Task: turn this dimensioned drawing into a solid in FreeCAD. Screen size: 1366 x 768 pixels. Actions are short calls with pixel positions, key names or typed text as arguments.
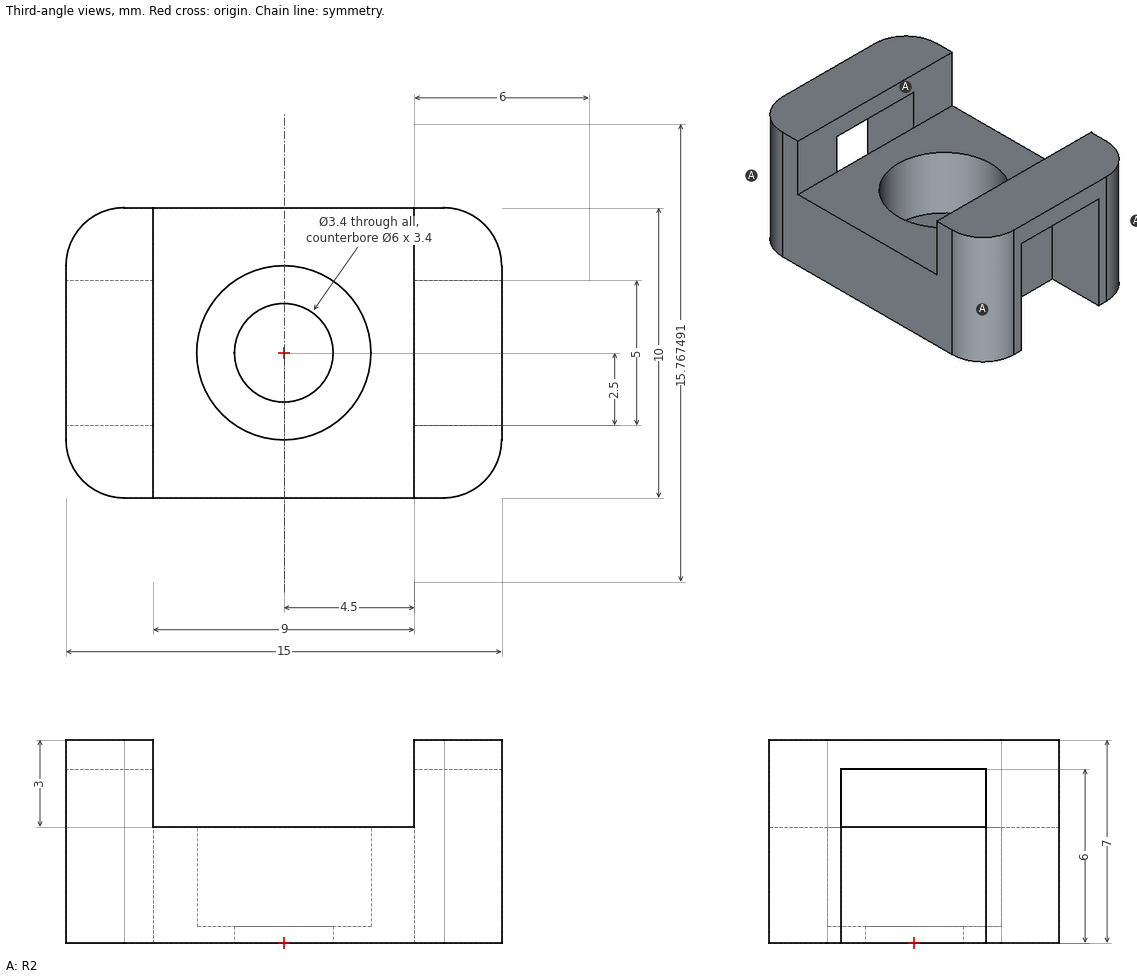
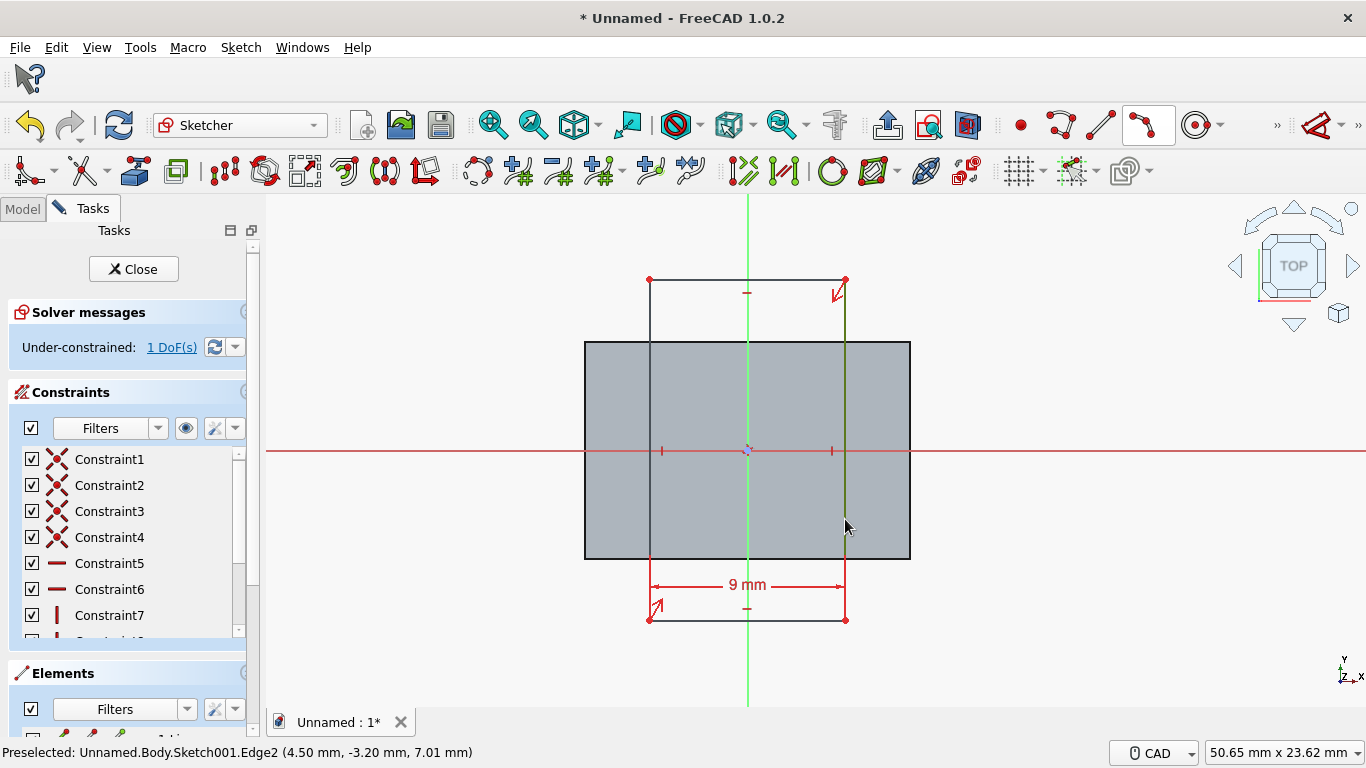
click(1344, 126)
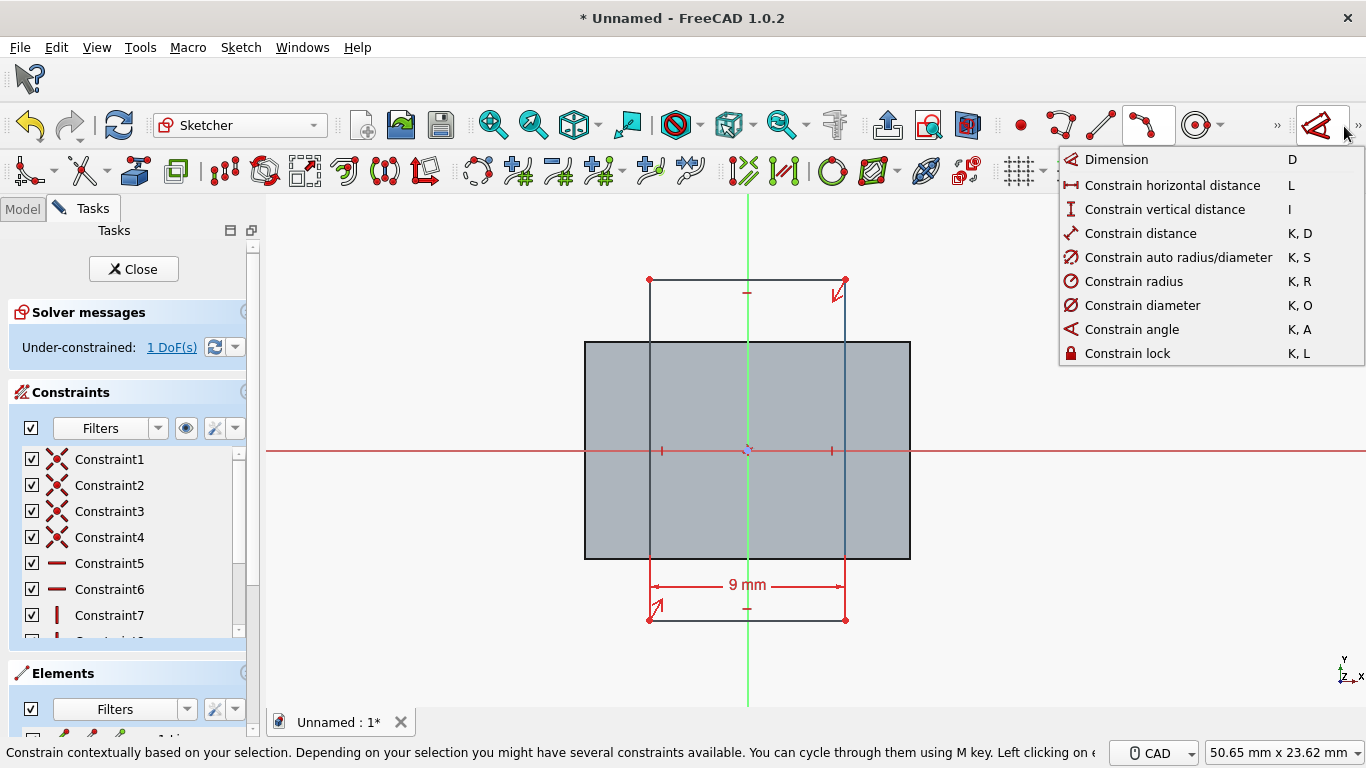
click(1212, 209)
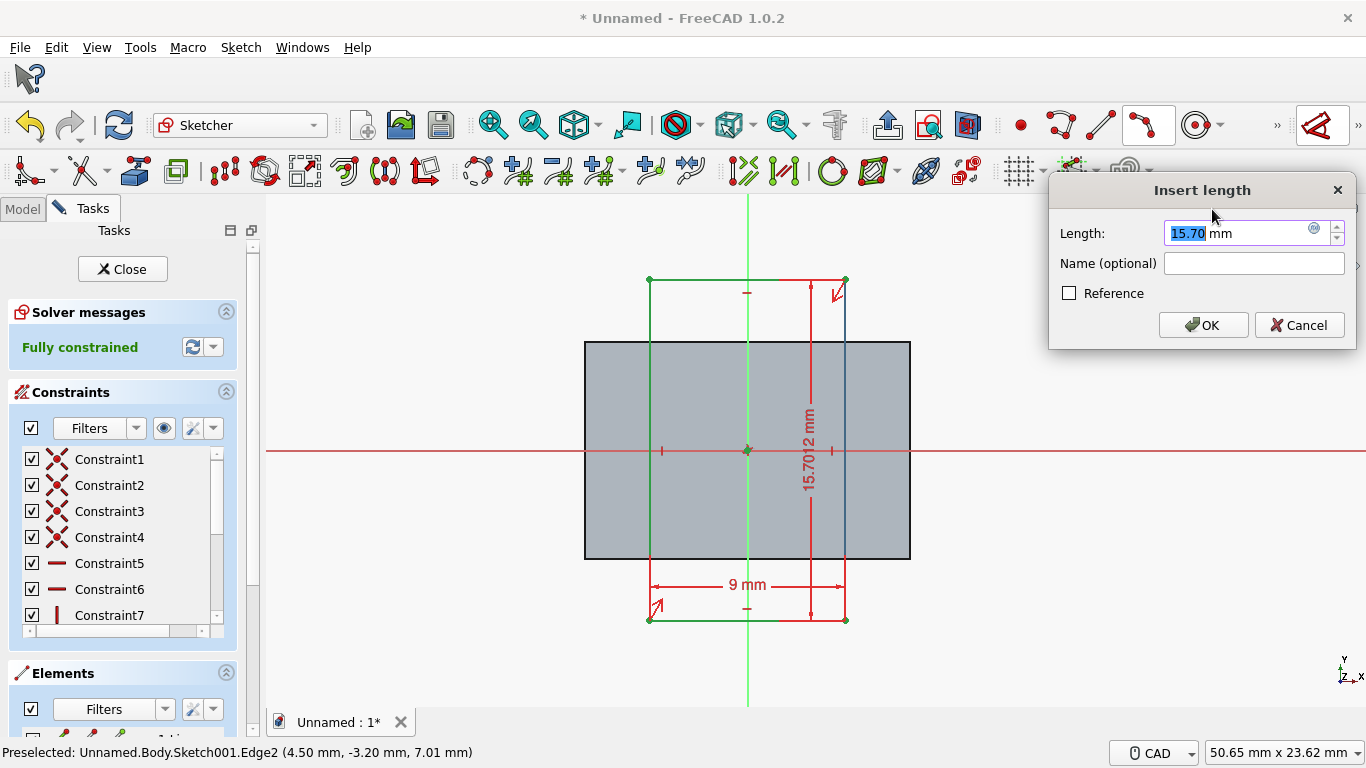
text(15.767491)
key(Return)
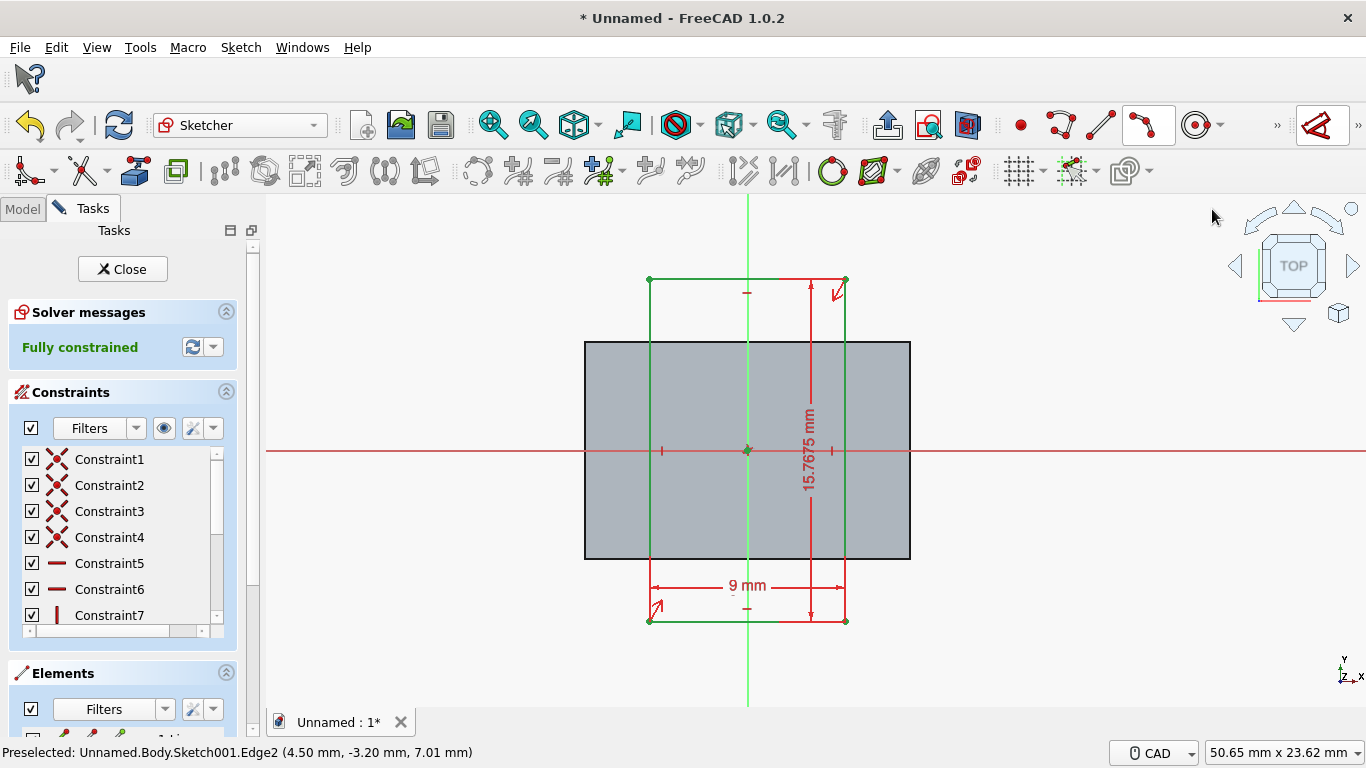
click(123, 269)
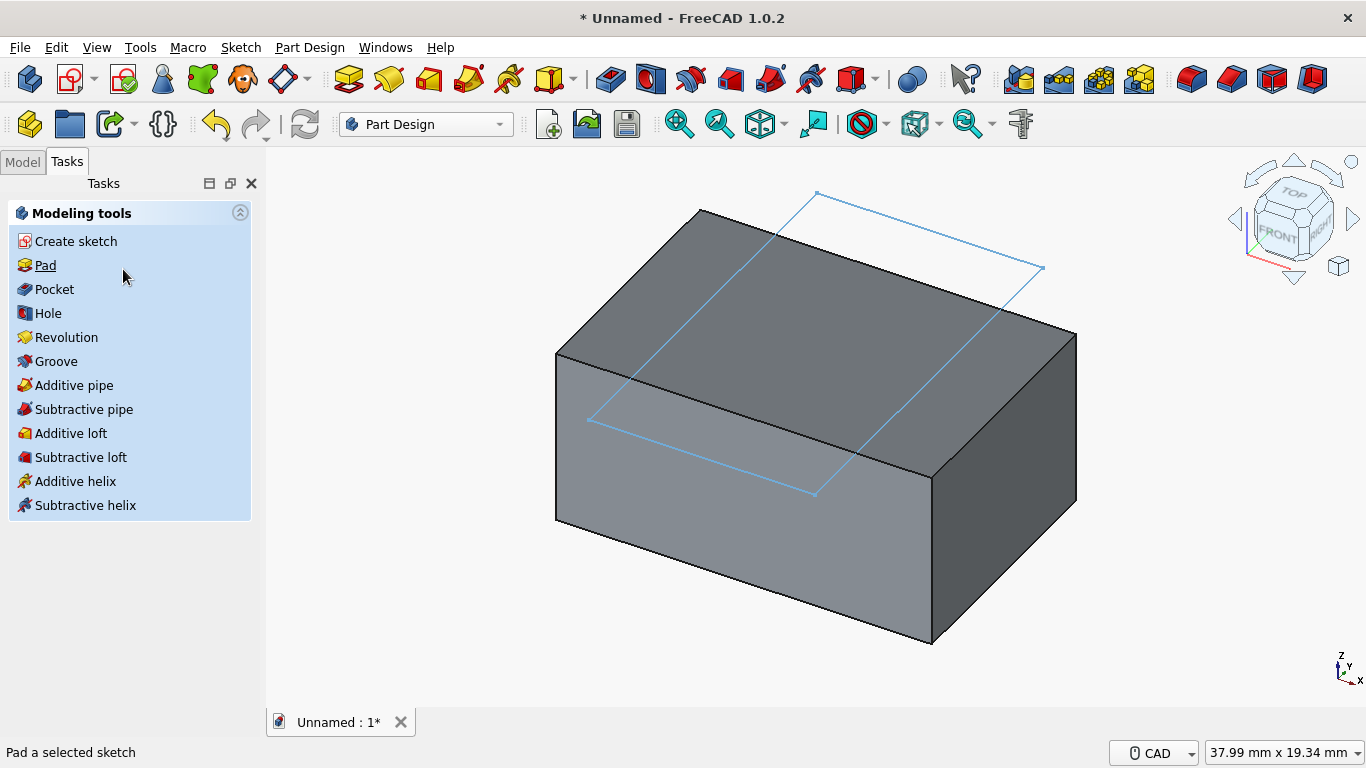
click(612, 80)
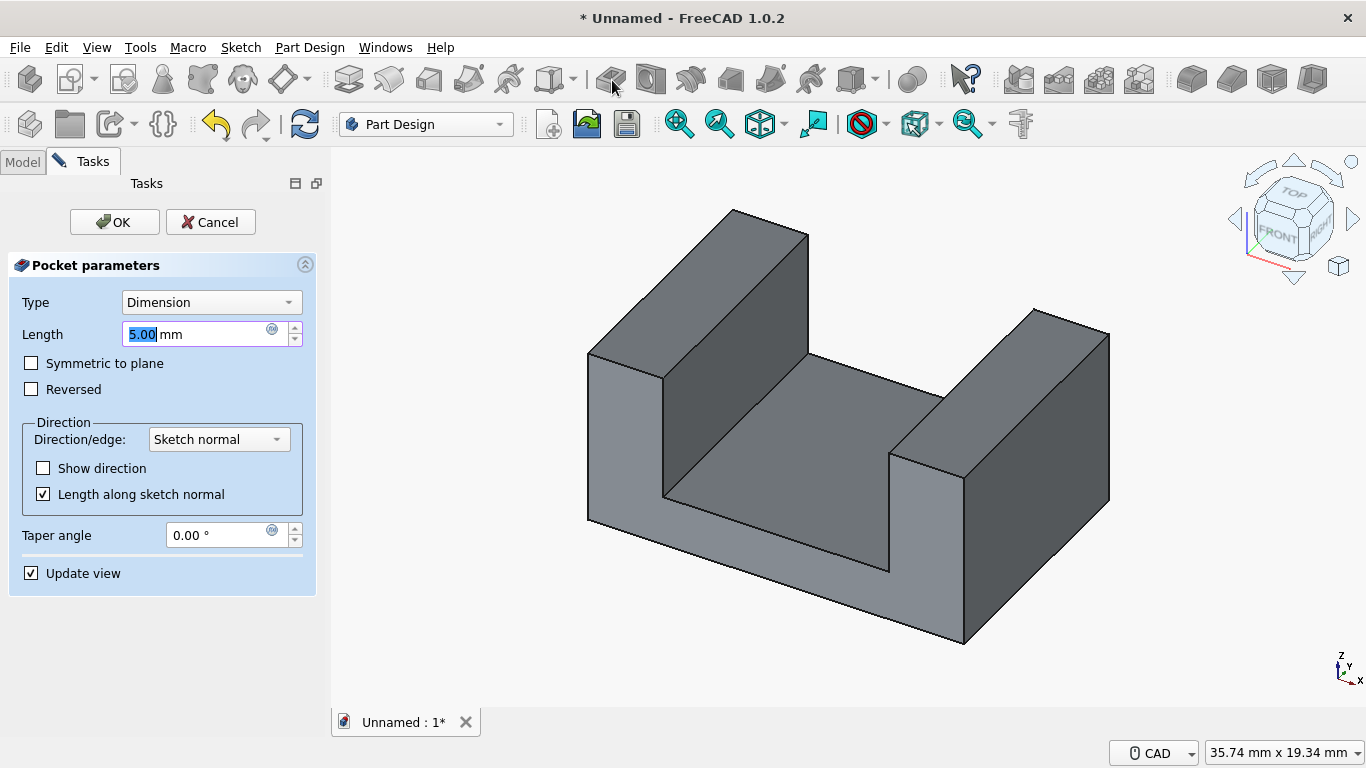
text(3)
key(Tab)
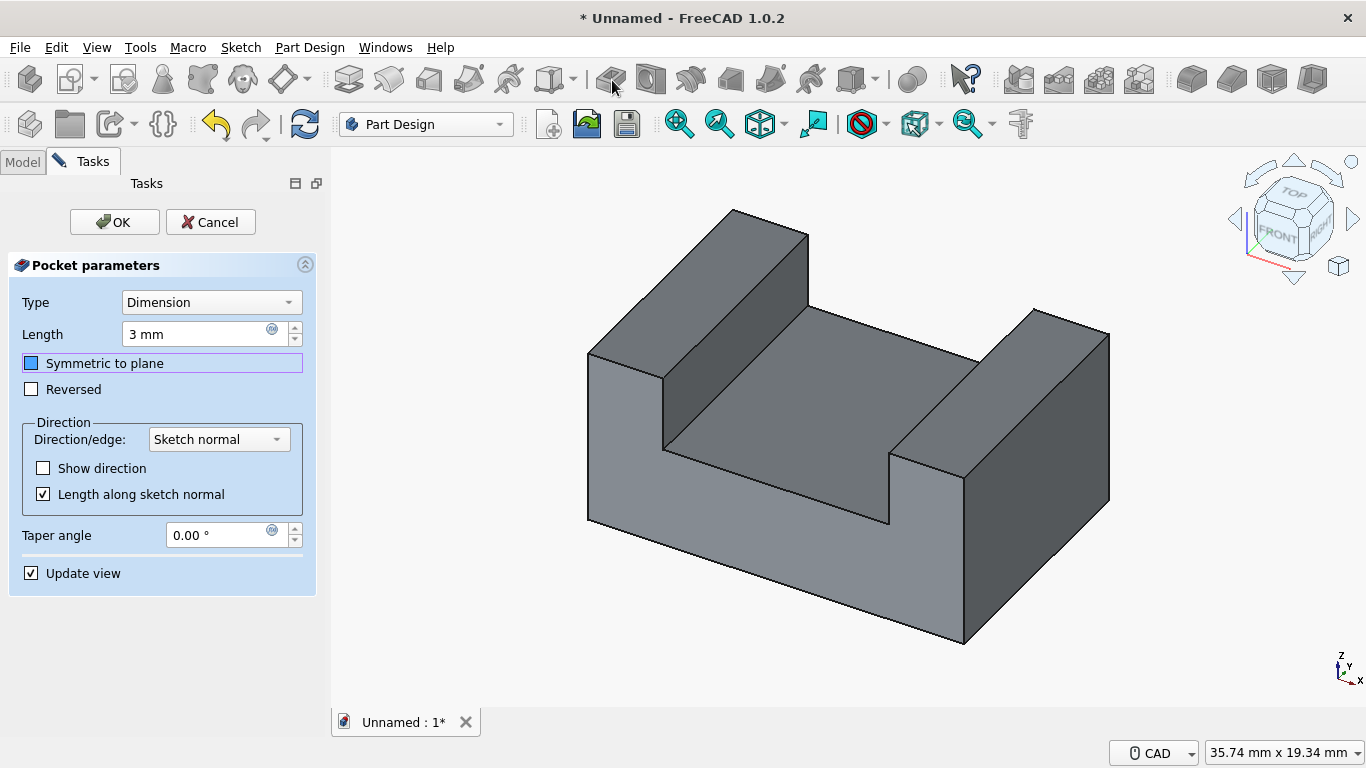
click(115, 222)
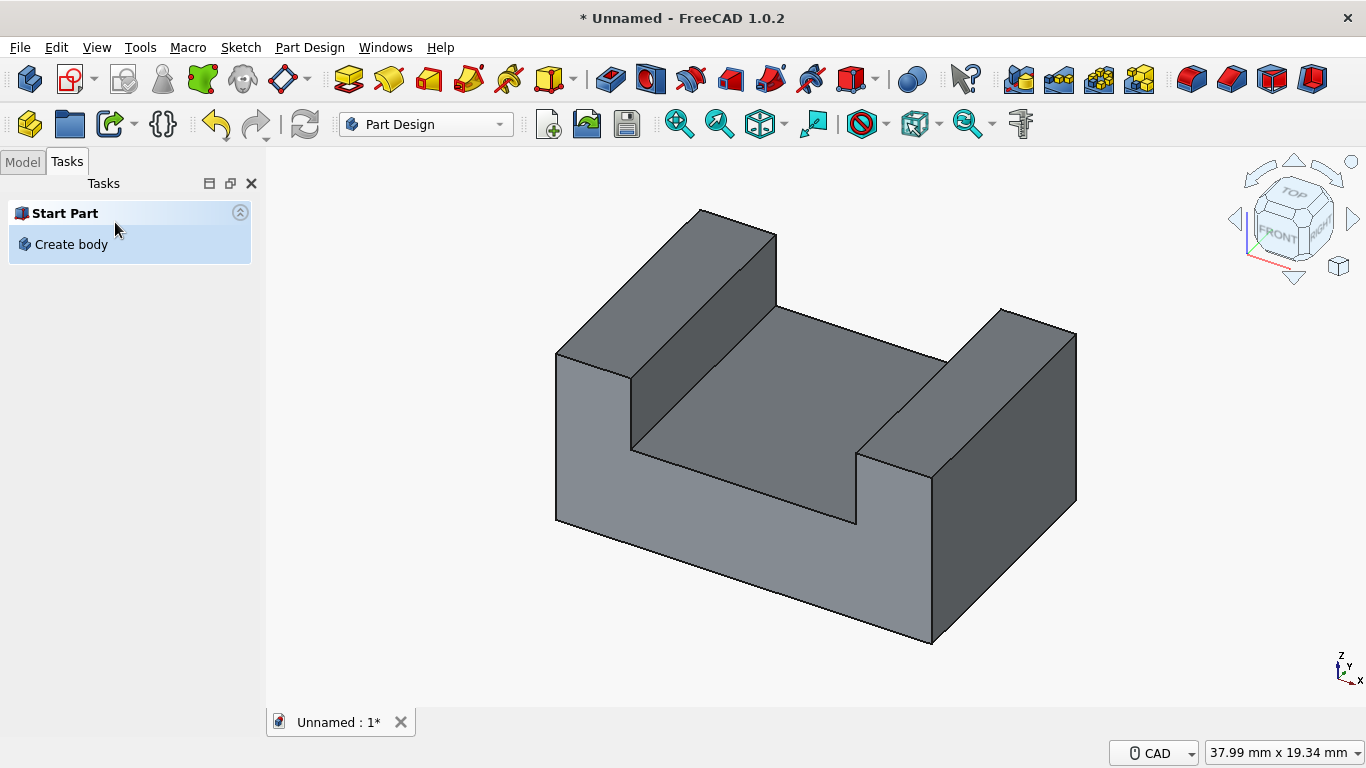
key(5)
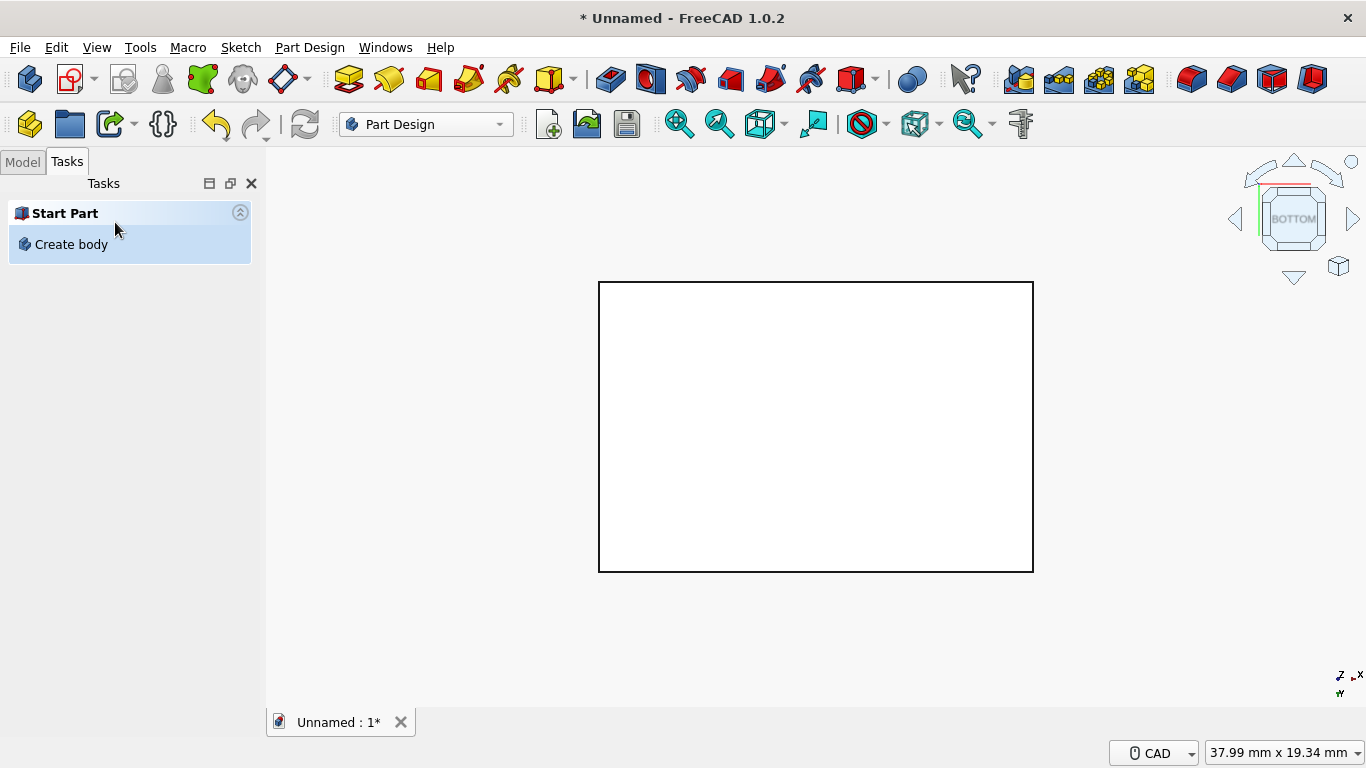
click(878, 426)